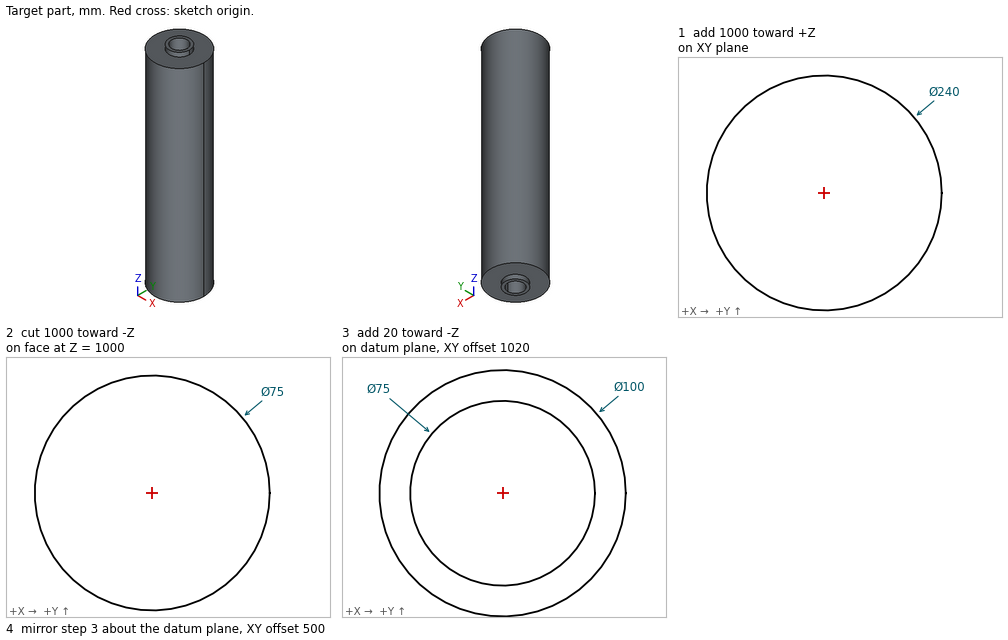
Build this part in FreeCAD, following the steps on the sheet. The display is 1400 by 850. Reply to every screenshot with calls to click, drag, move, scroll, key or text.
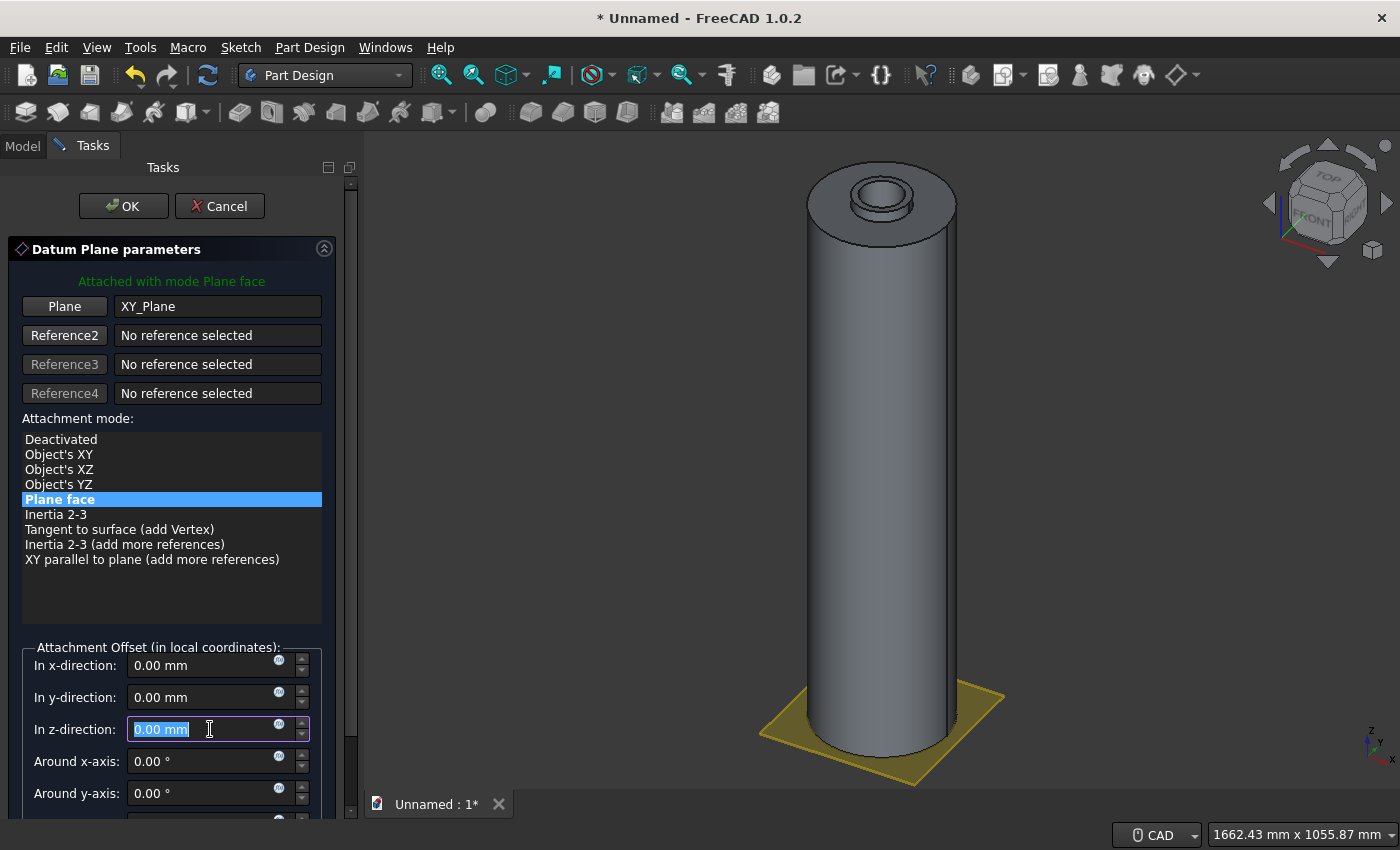
text(500)
key(Tab)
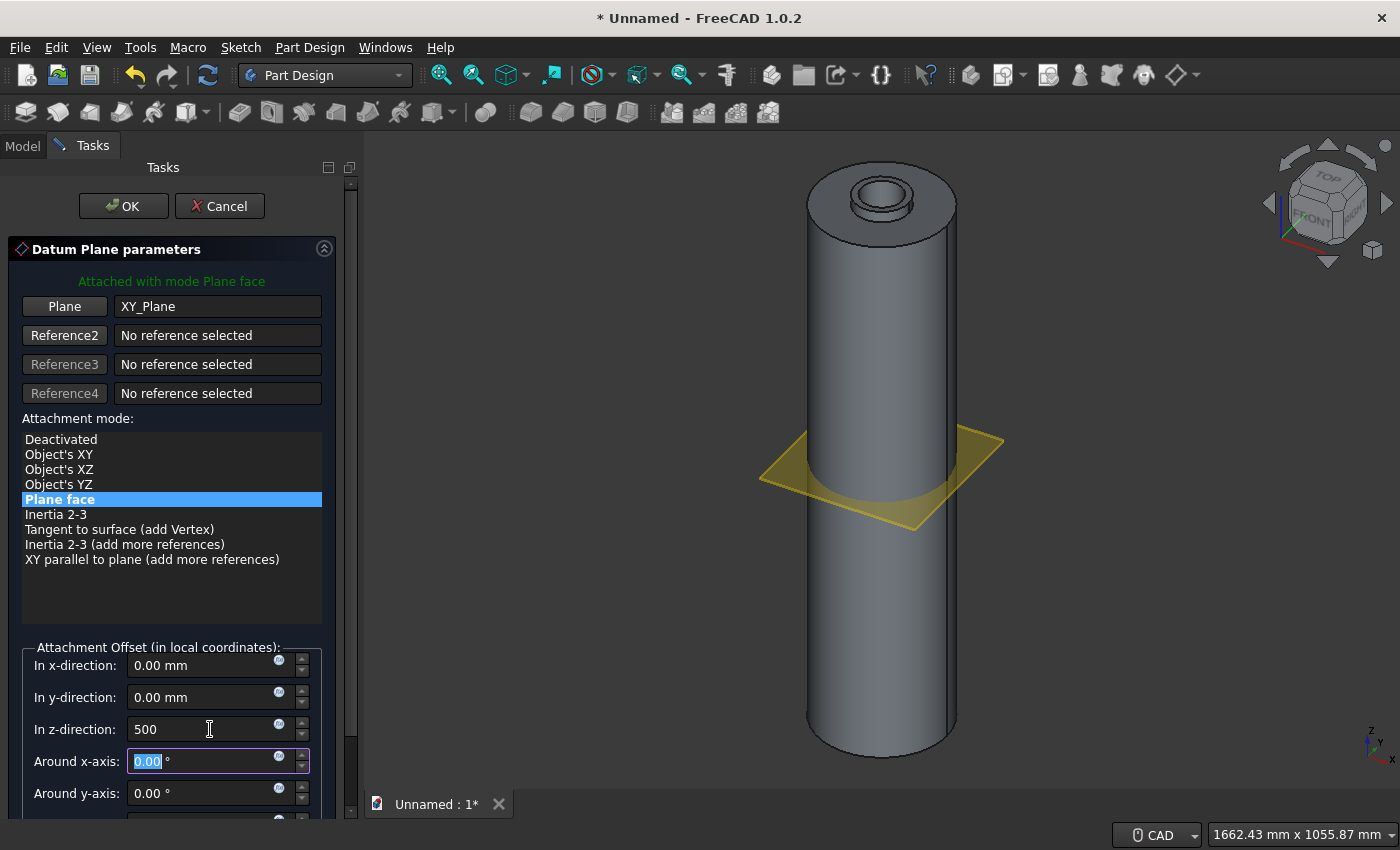
click(124, 206)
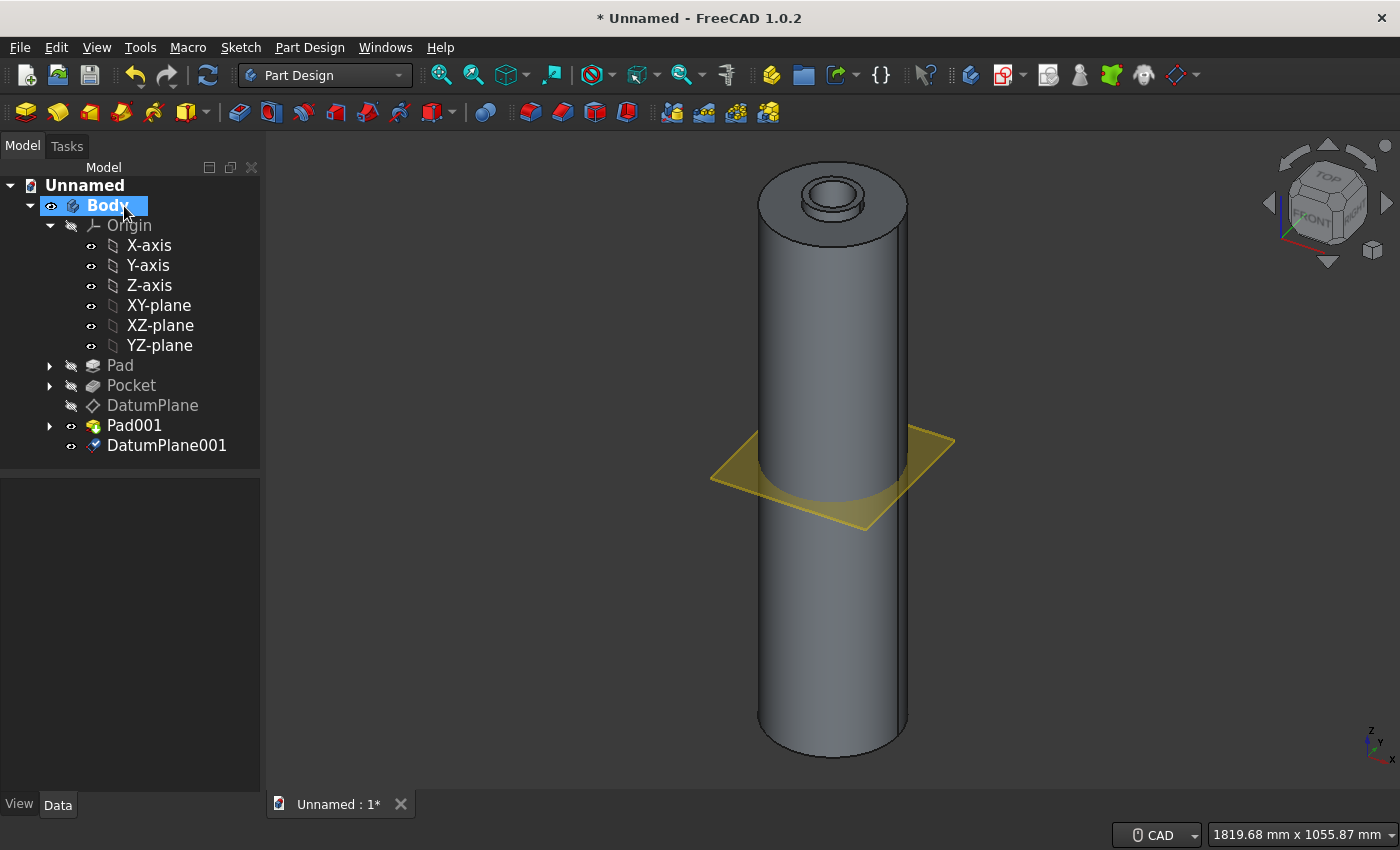
click(116, 426)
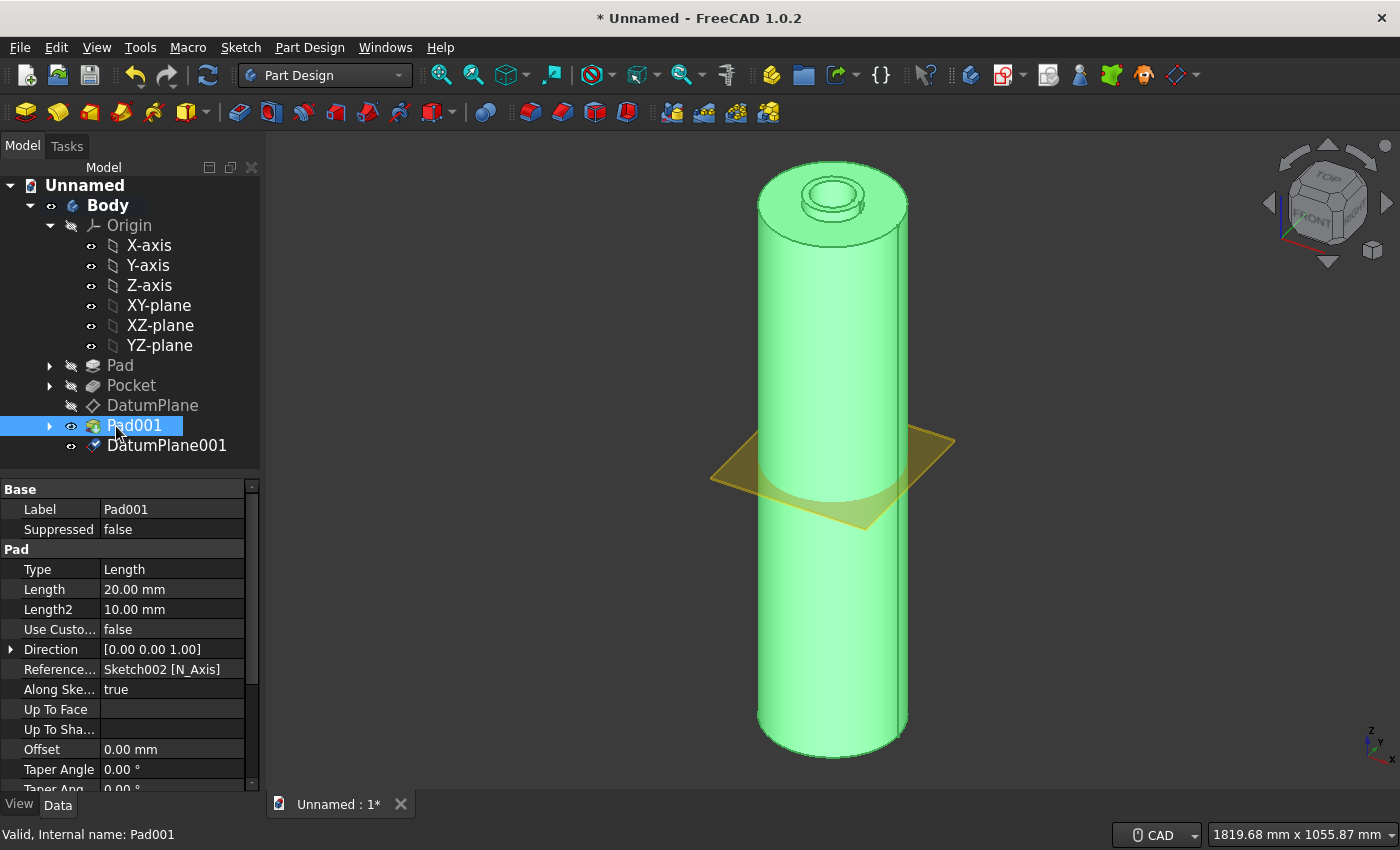
click(672, 112)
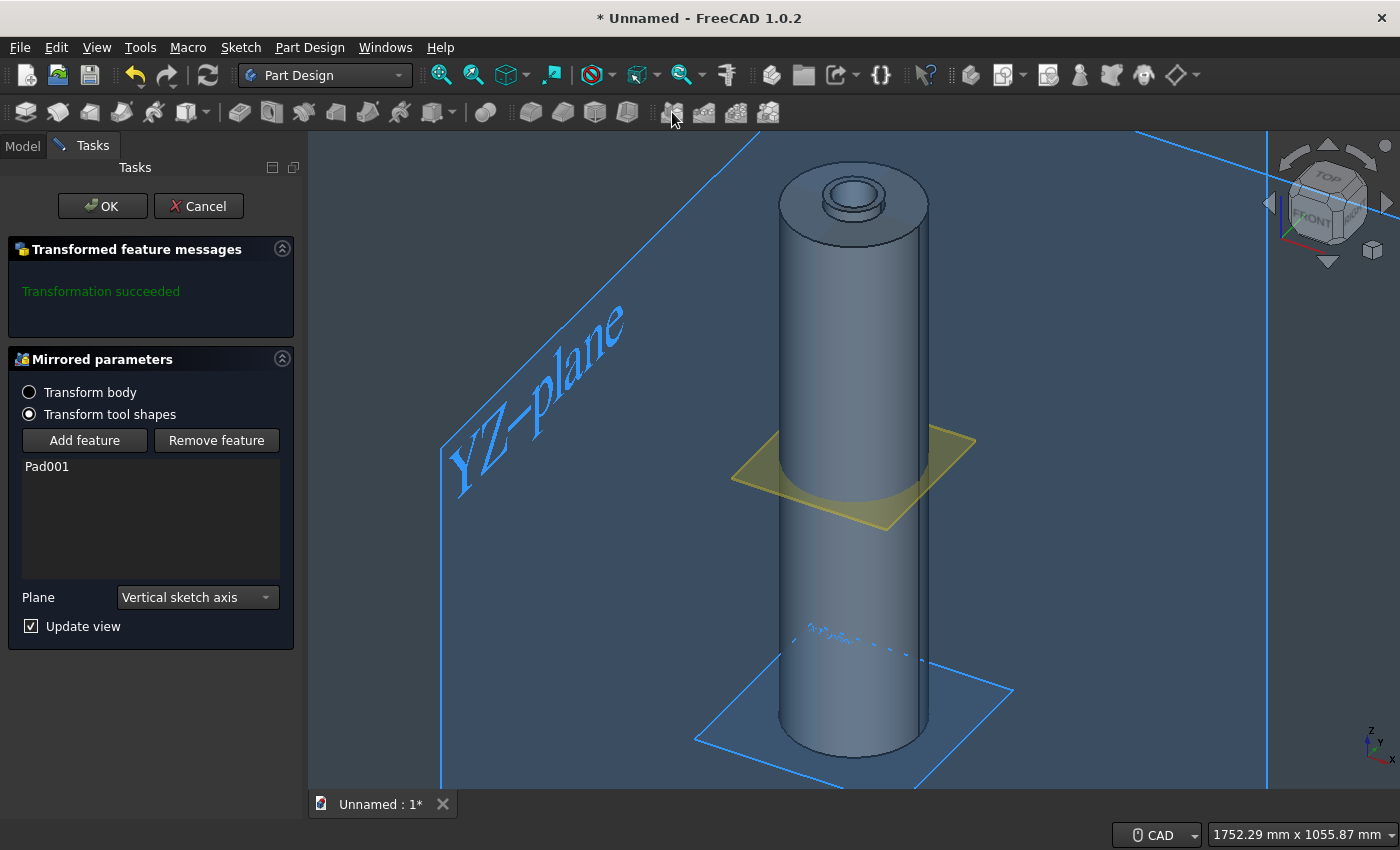
click(198, 598)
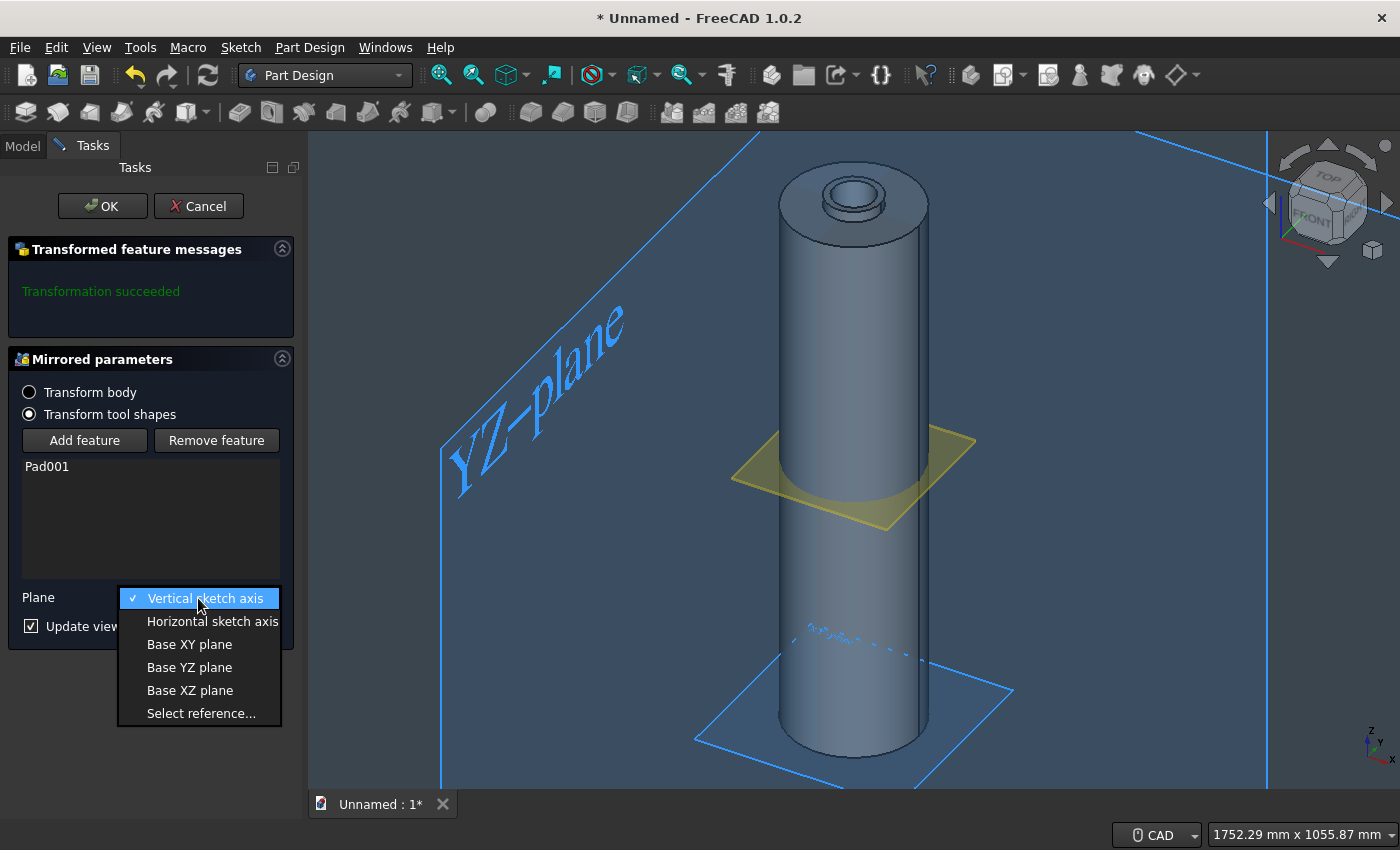
click(198, 714)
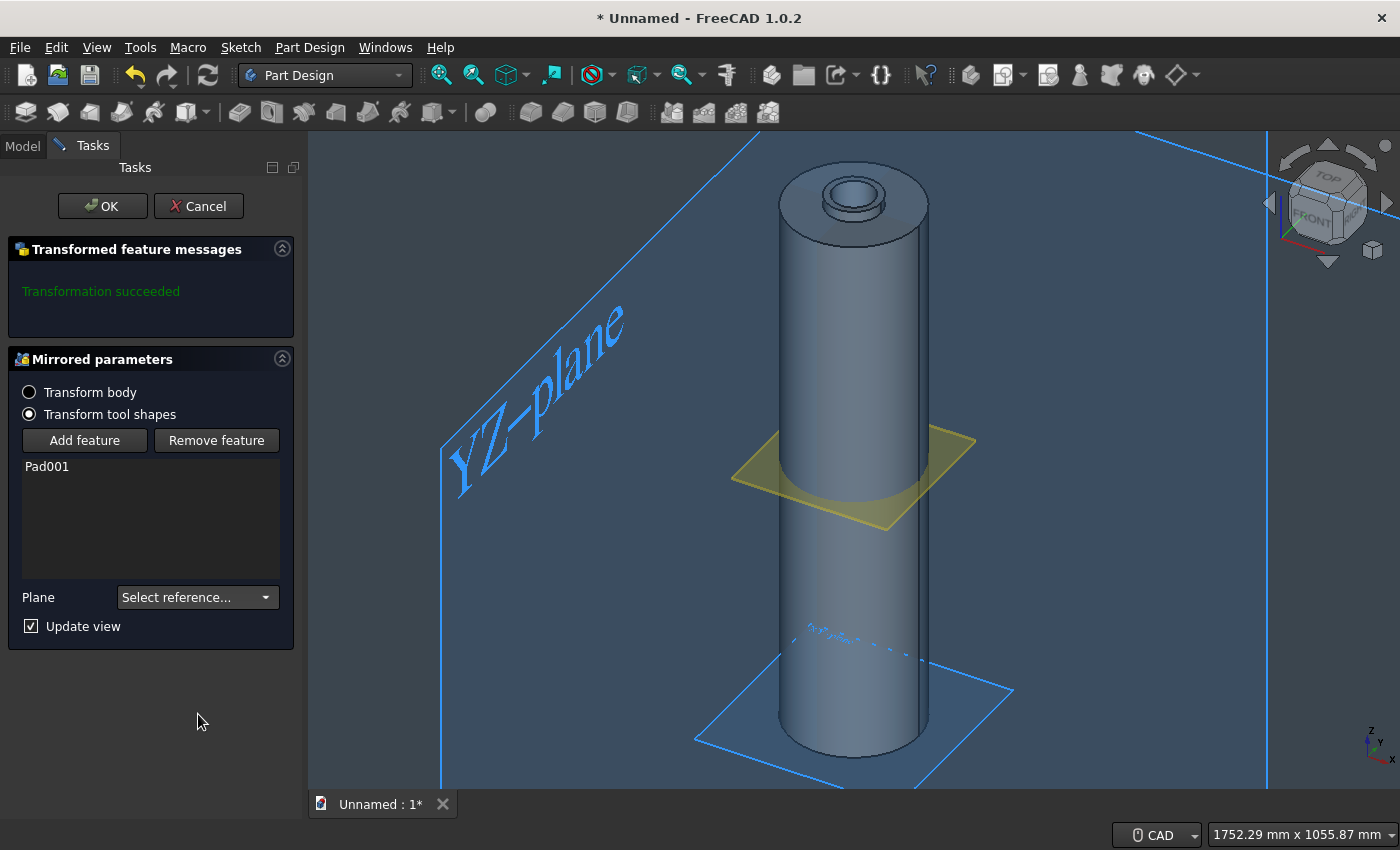
click(23, 145)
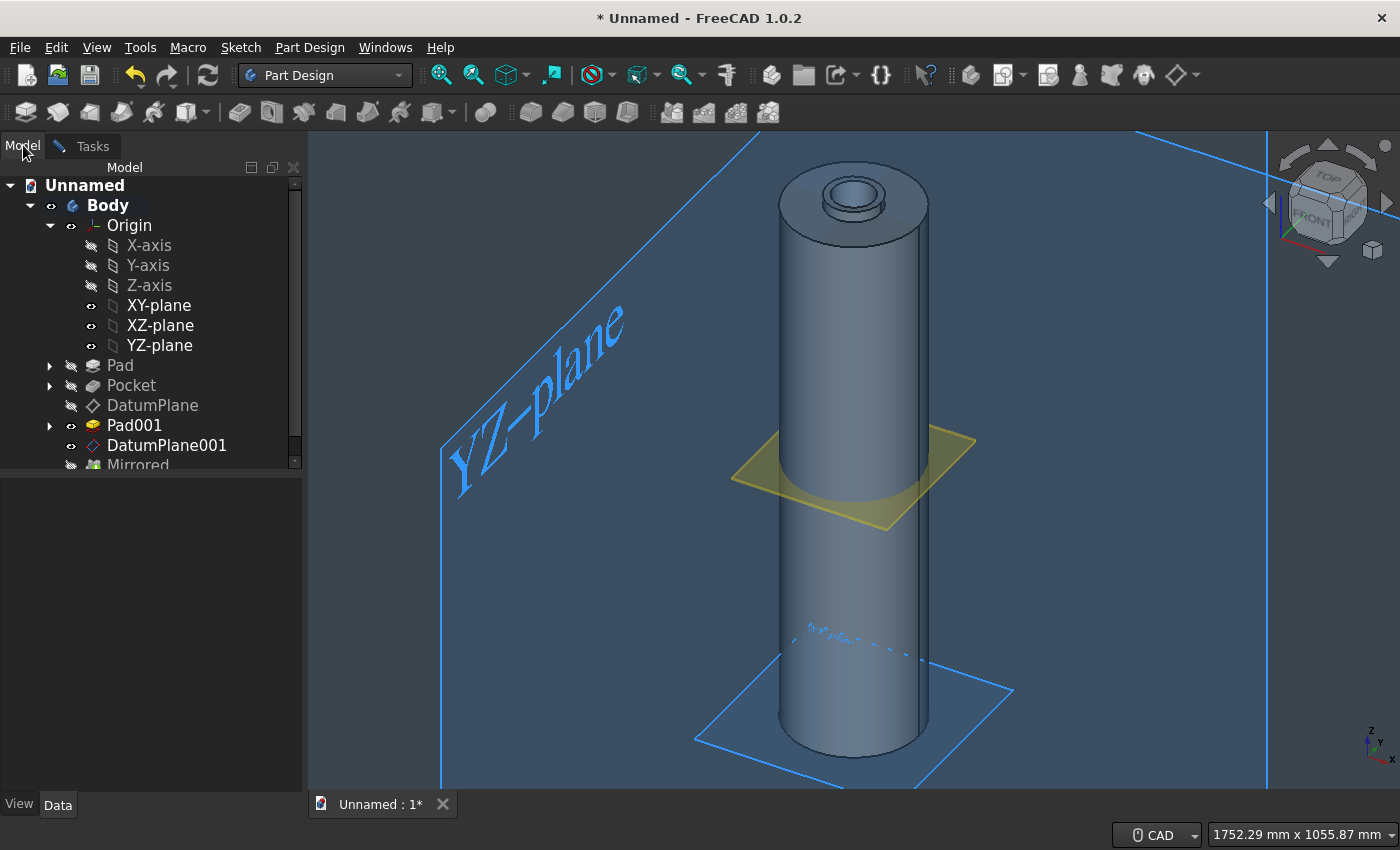
click(116, 446)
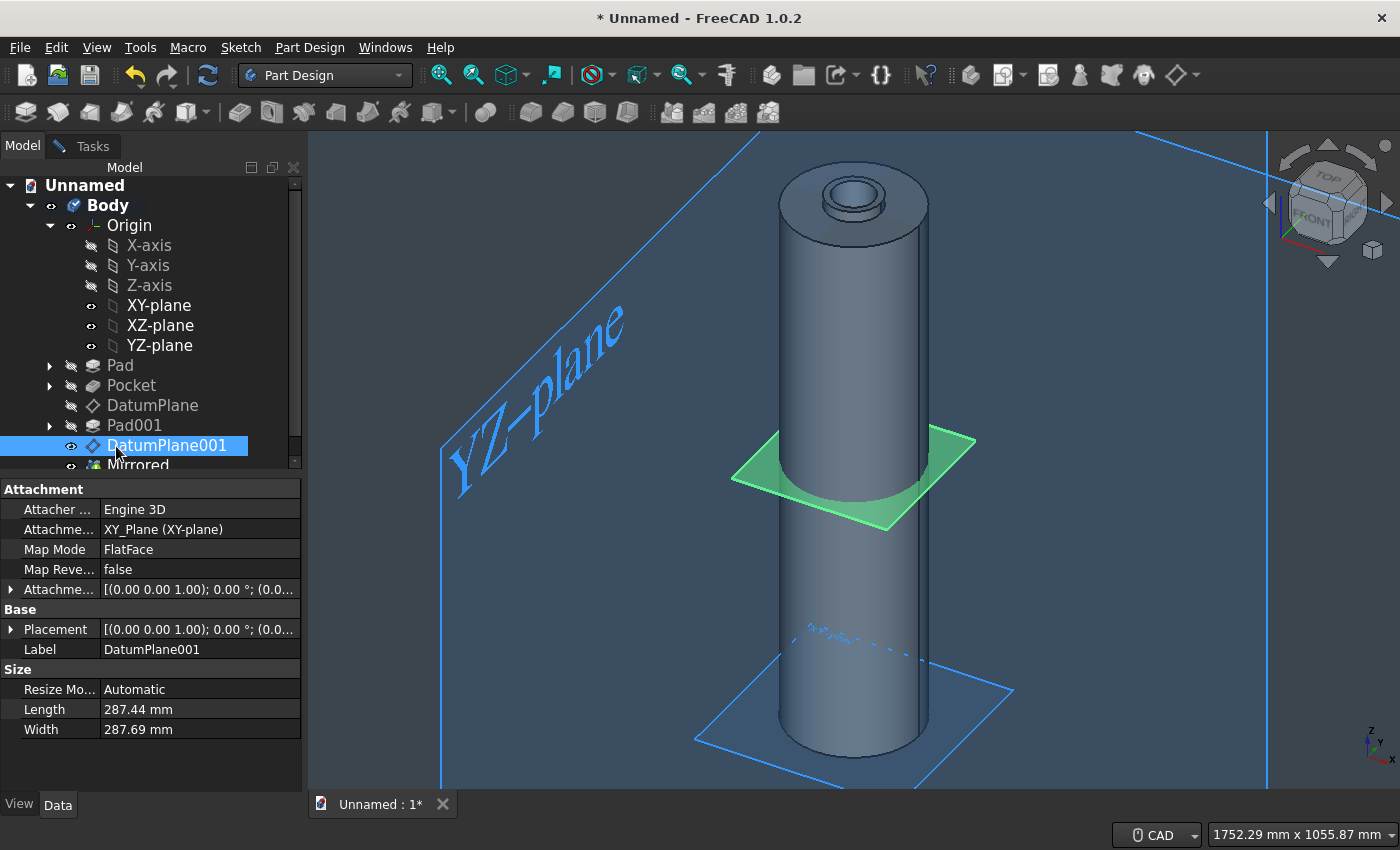
click(84, 145)